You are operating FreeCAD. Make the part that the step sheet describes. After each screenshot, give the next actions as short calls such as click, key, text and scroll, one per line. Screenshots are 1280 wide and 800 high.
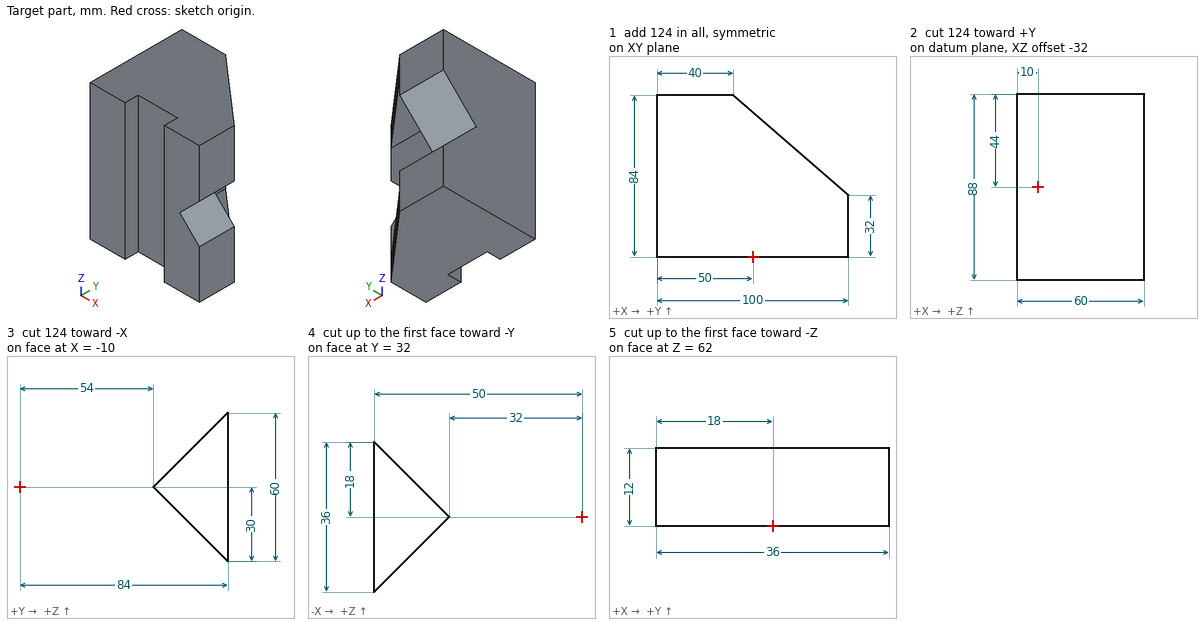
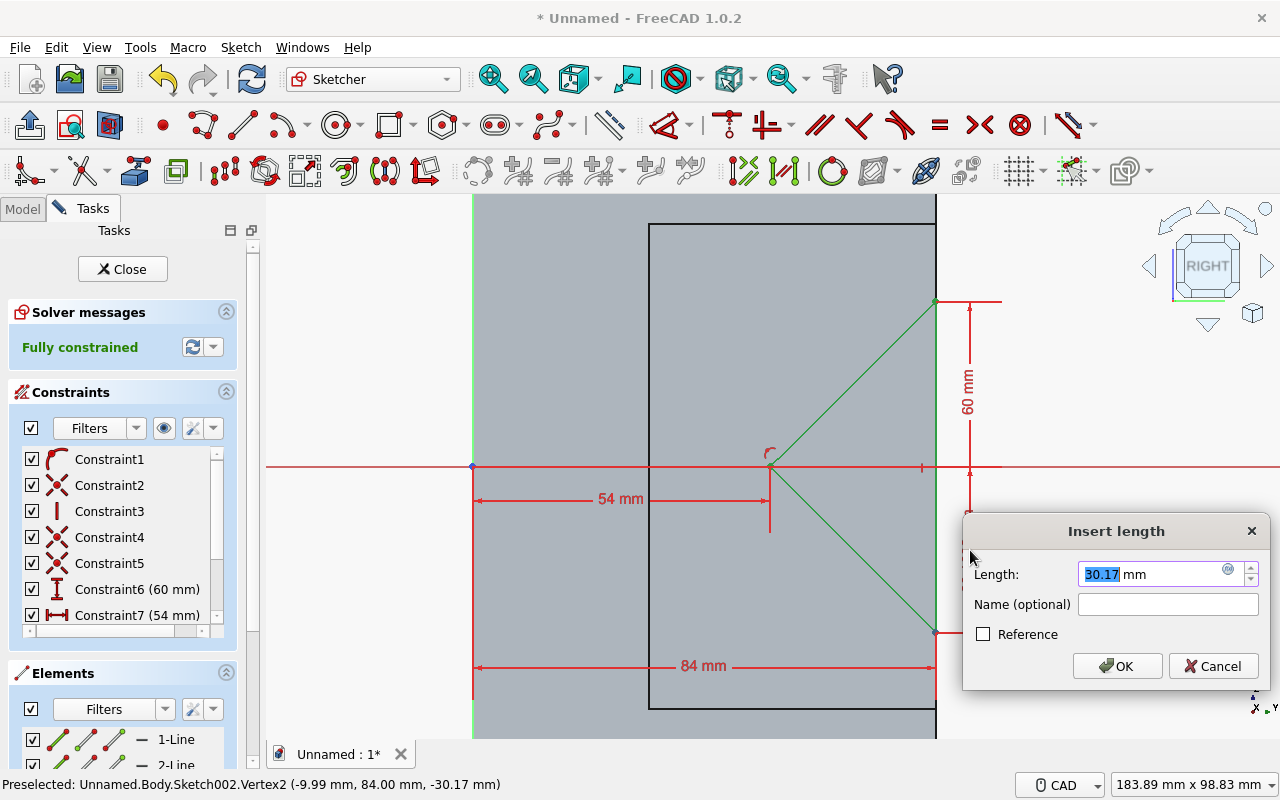
text(30)
key(Return)
key(Escape)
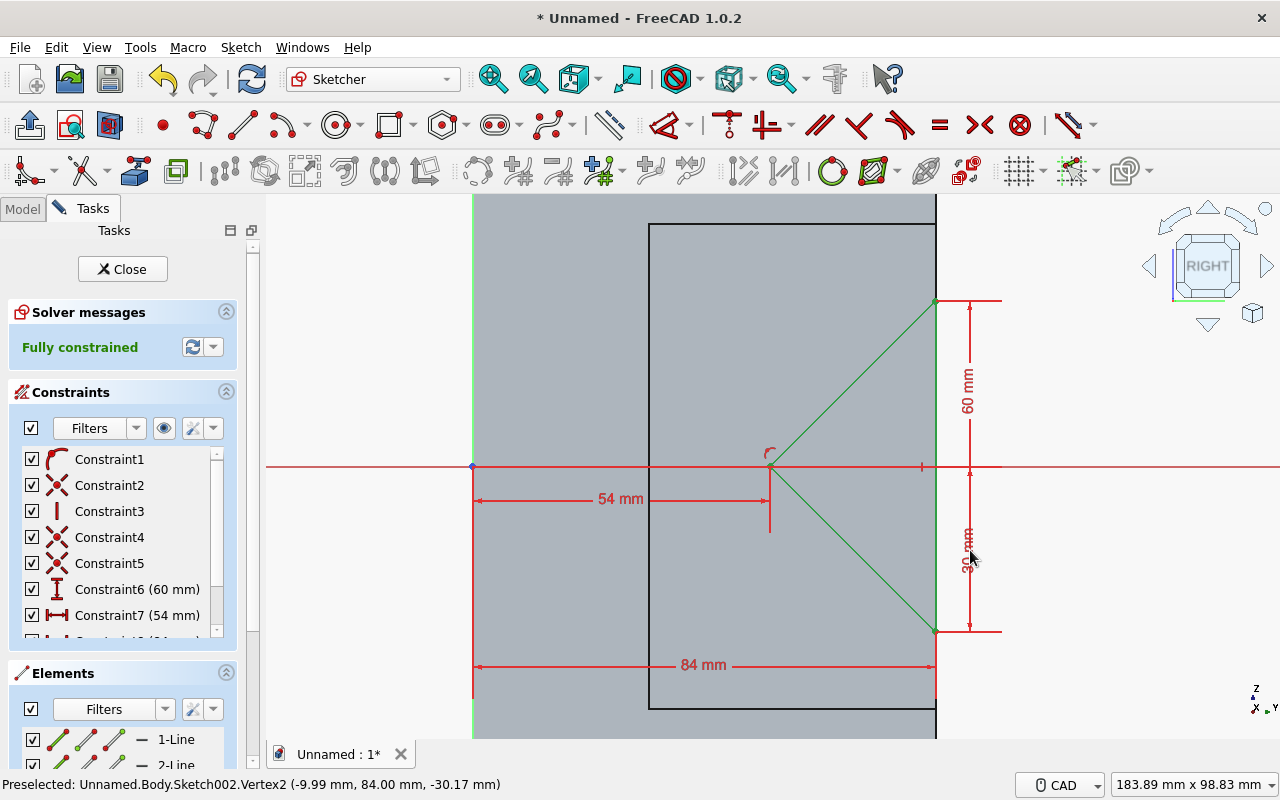
click(123, 269)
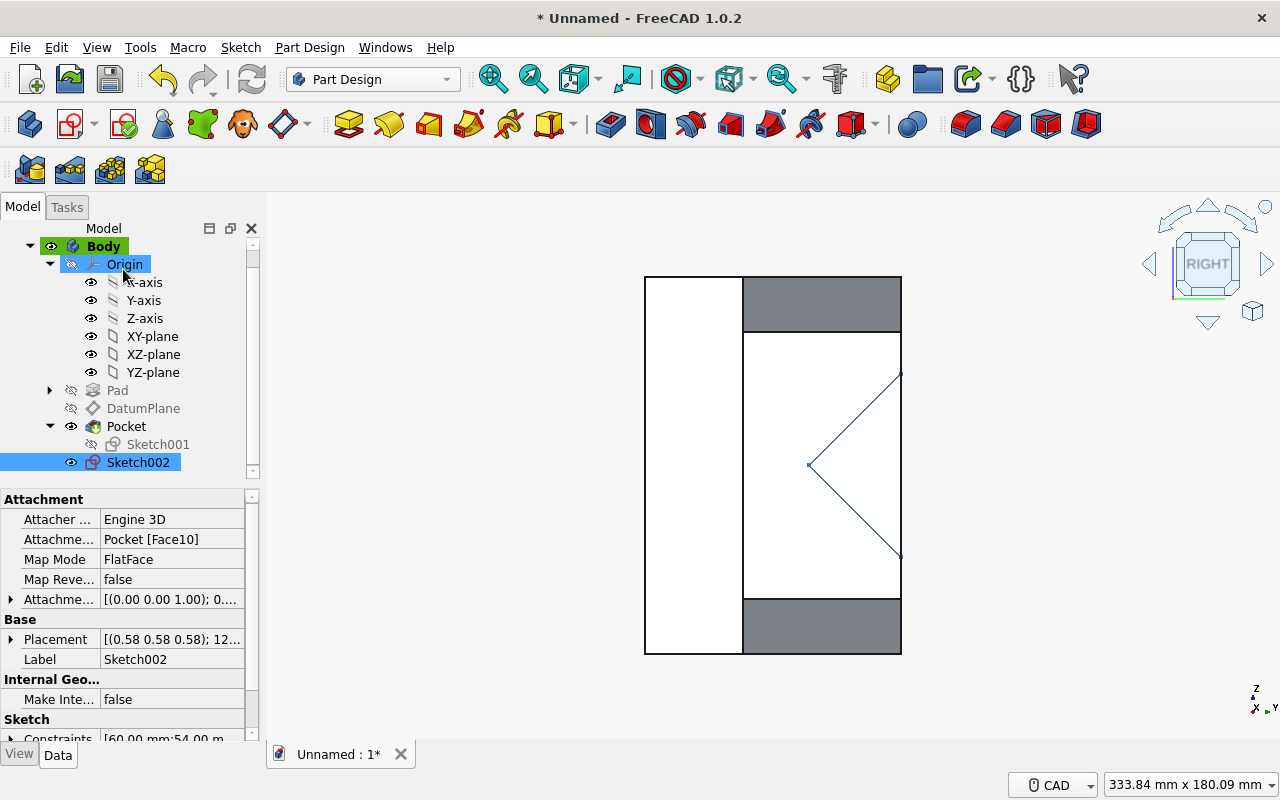
click(612, 124)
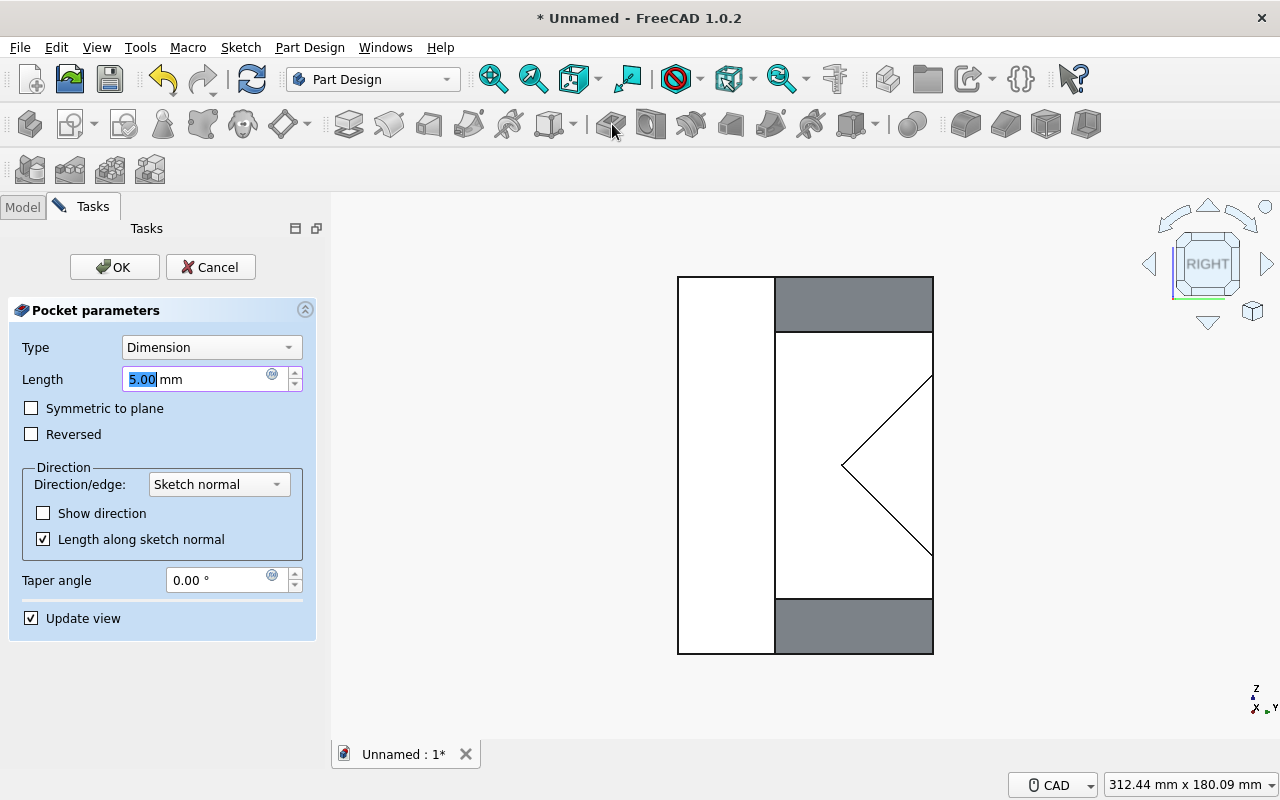
text(124)
key(Tab)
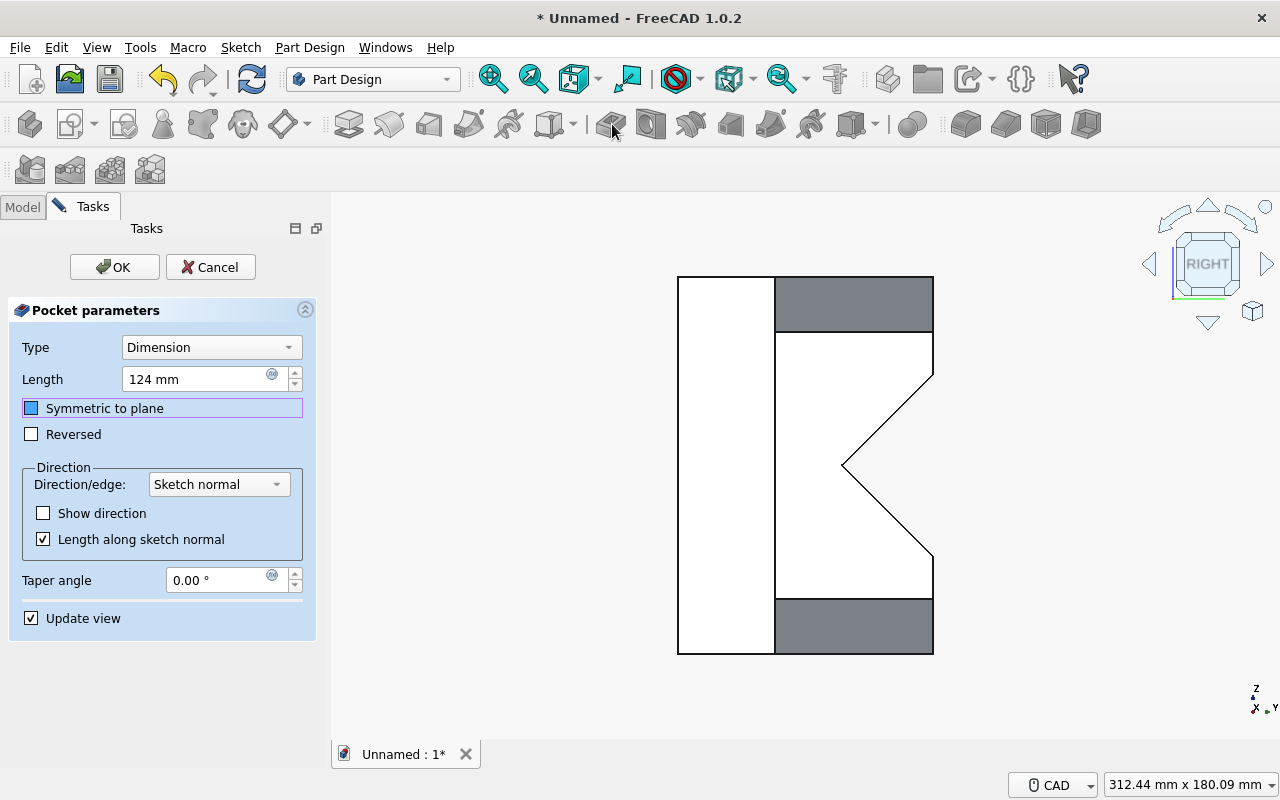
click(115, 267)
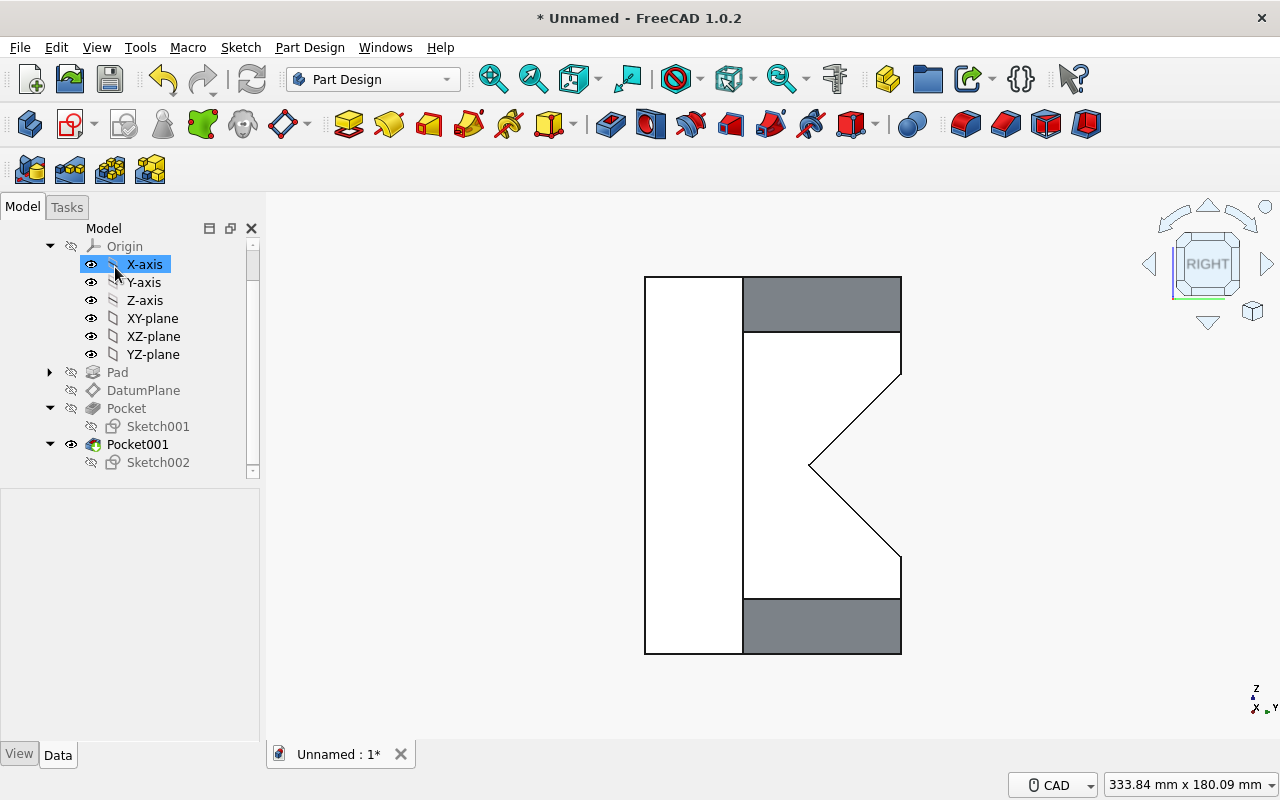
key(4)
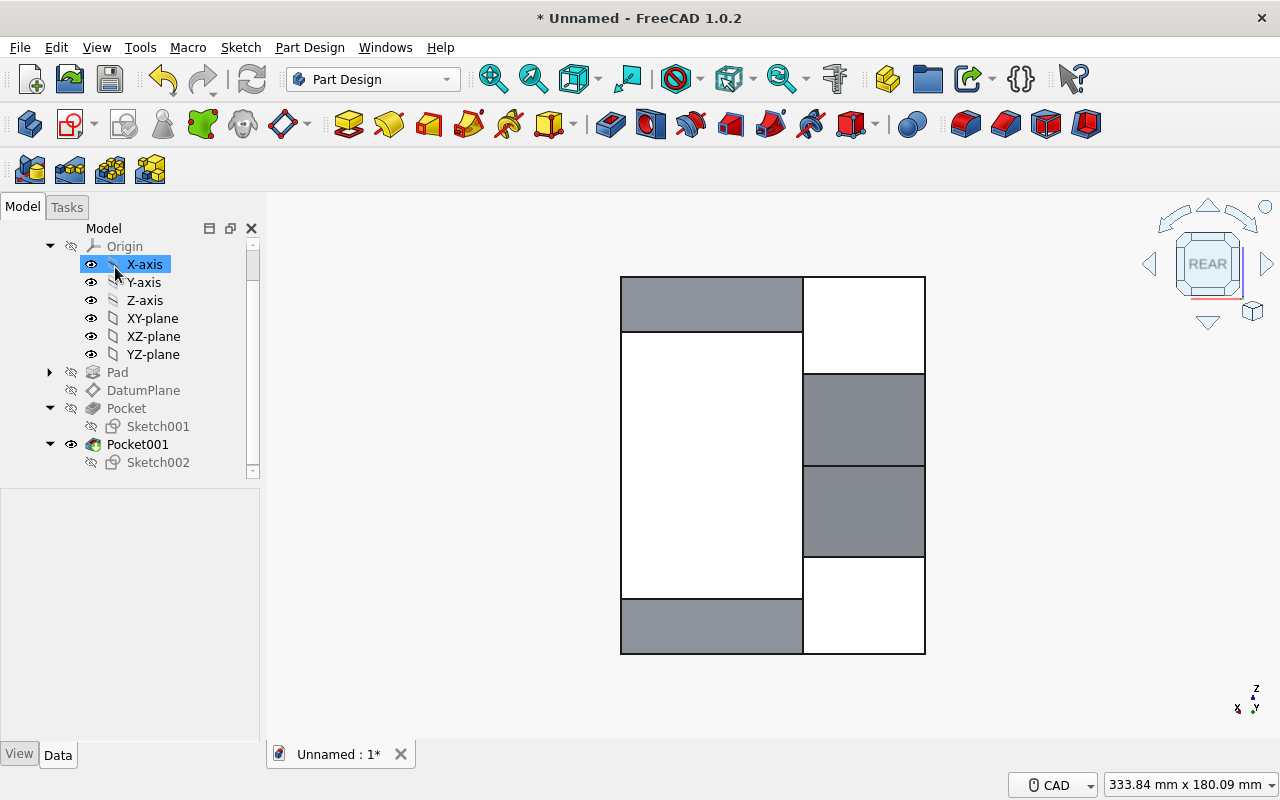
click(712, 426)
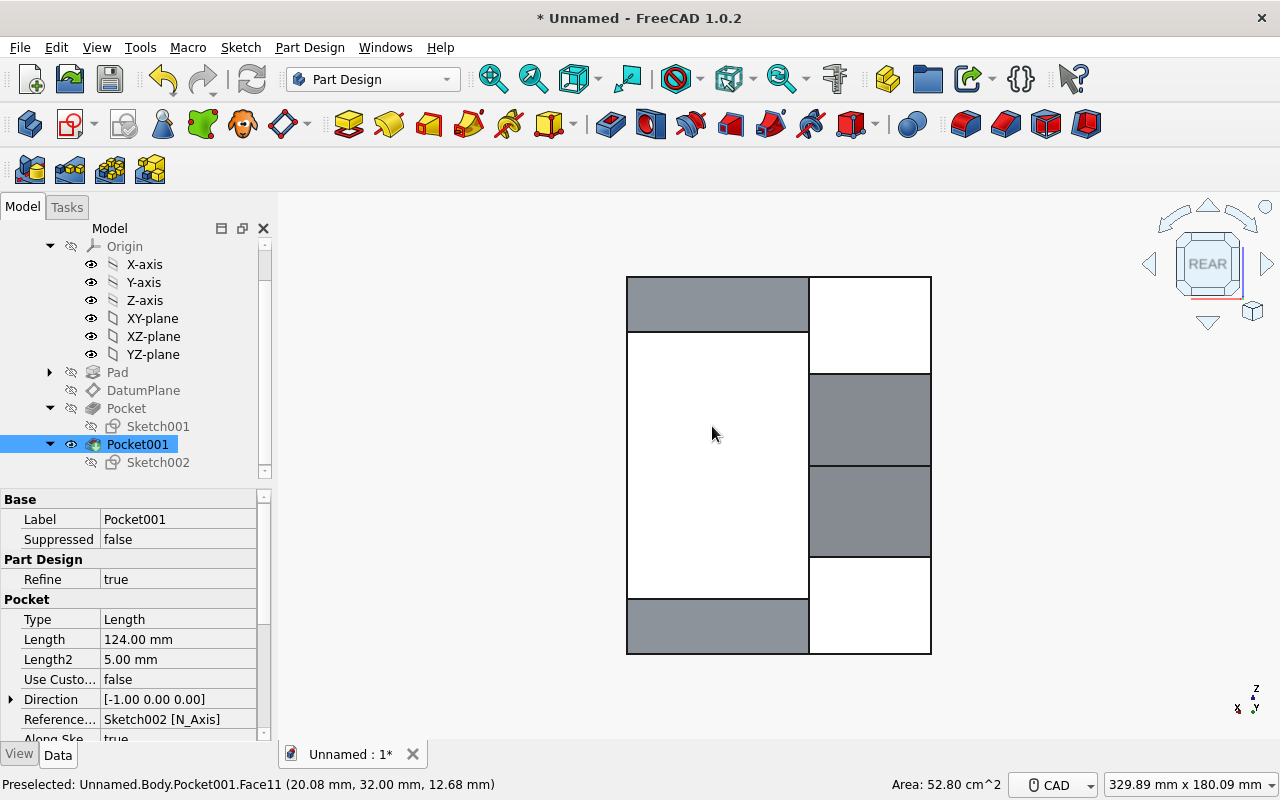
click(70, 124)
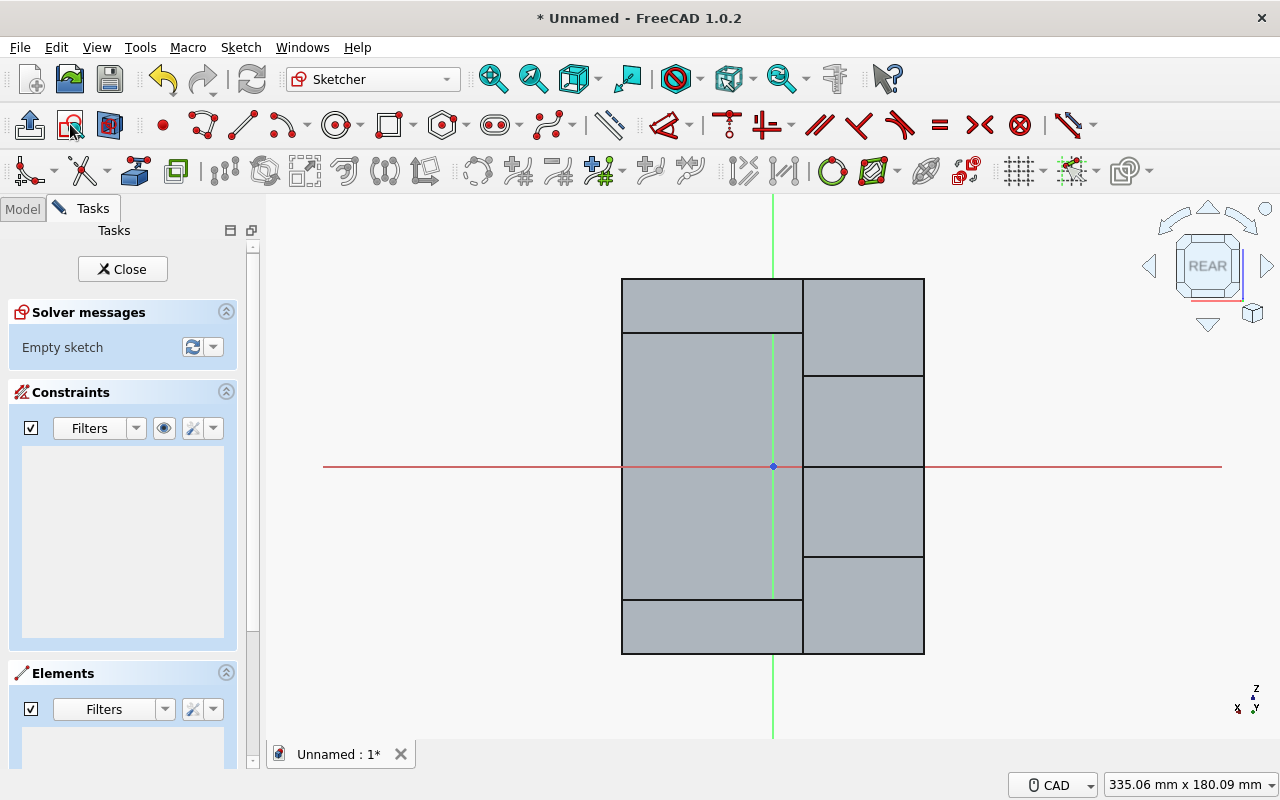
scroll(694, 467, up, 6)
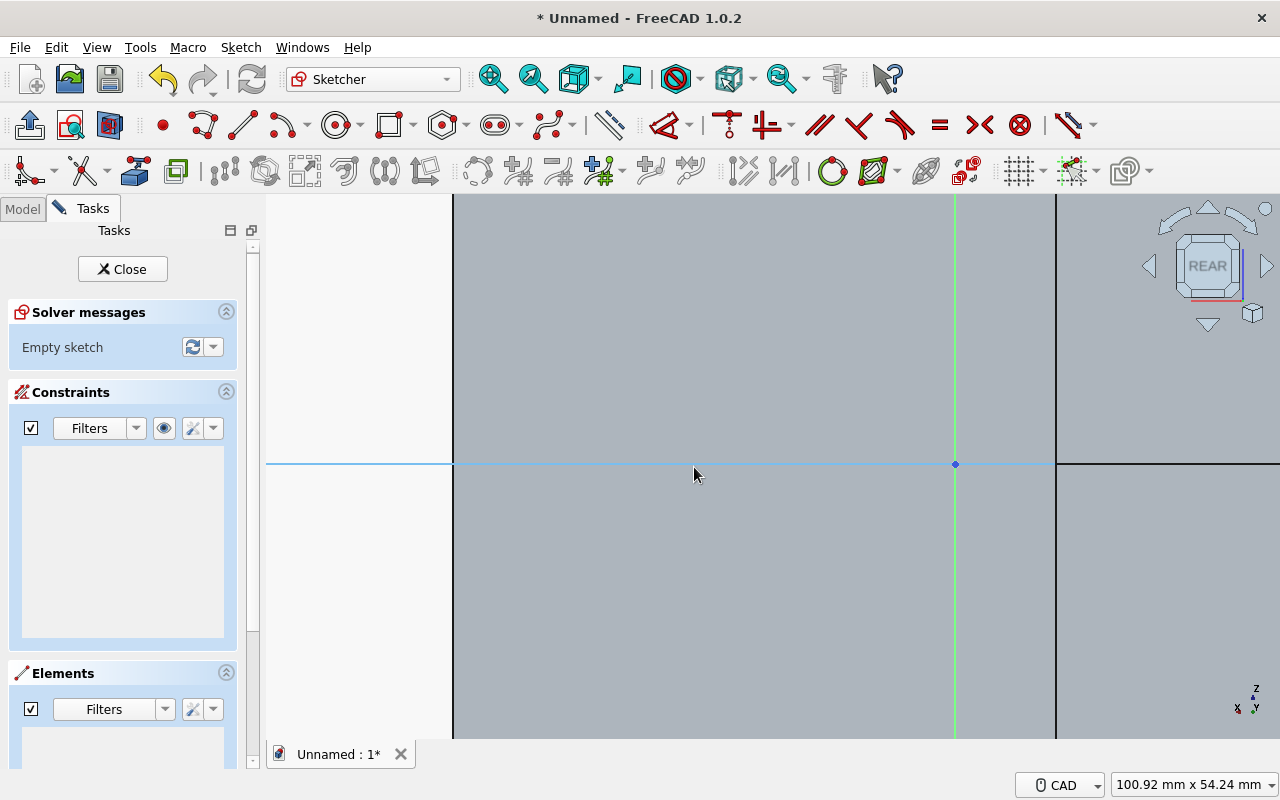
click(204, 126)